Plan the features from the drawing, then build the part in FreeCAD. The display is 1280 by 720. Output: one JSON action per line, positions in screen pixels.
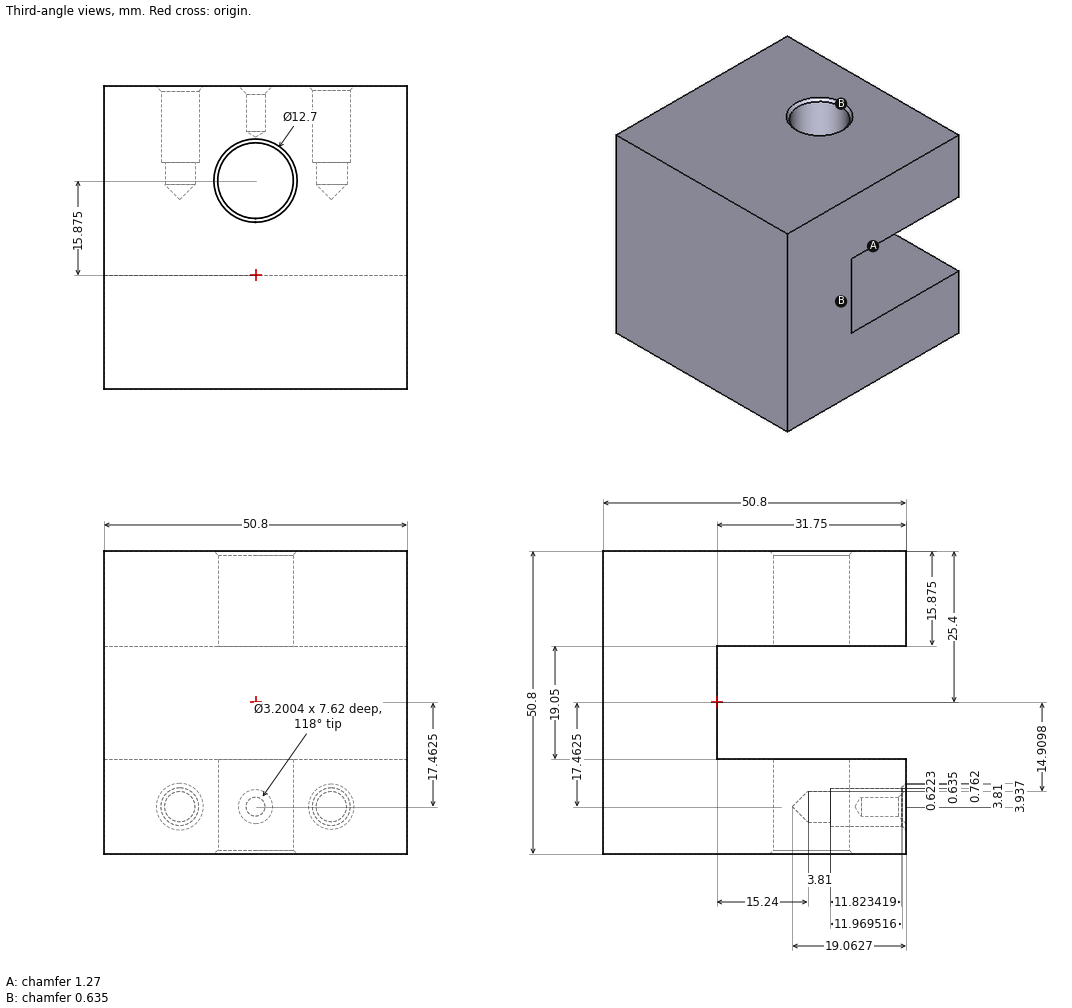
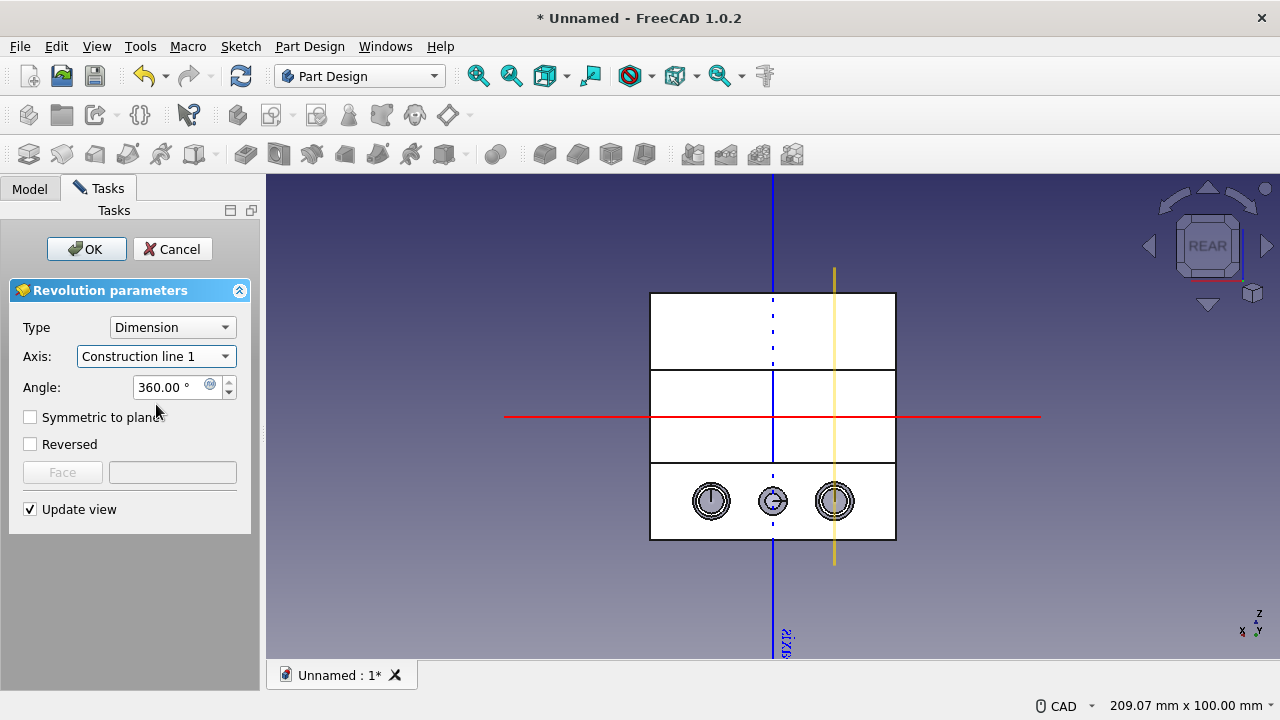
{"action": "left_click", "coordinate": [87, 249]}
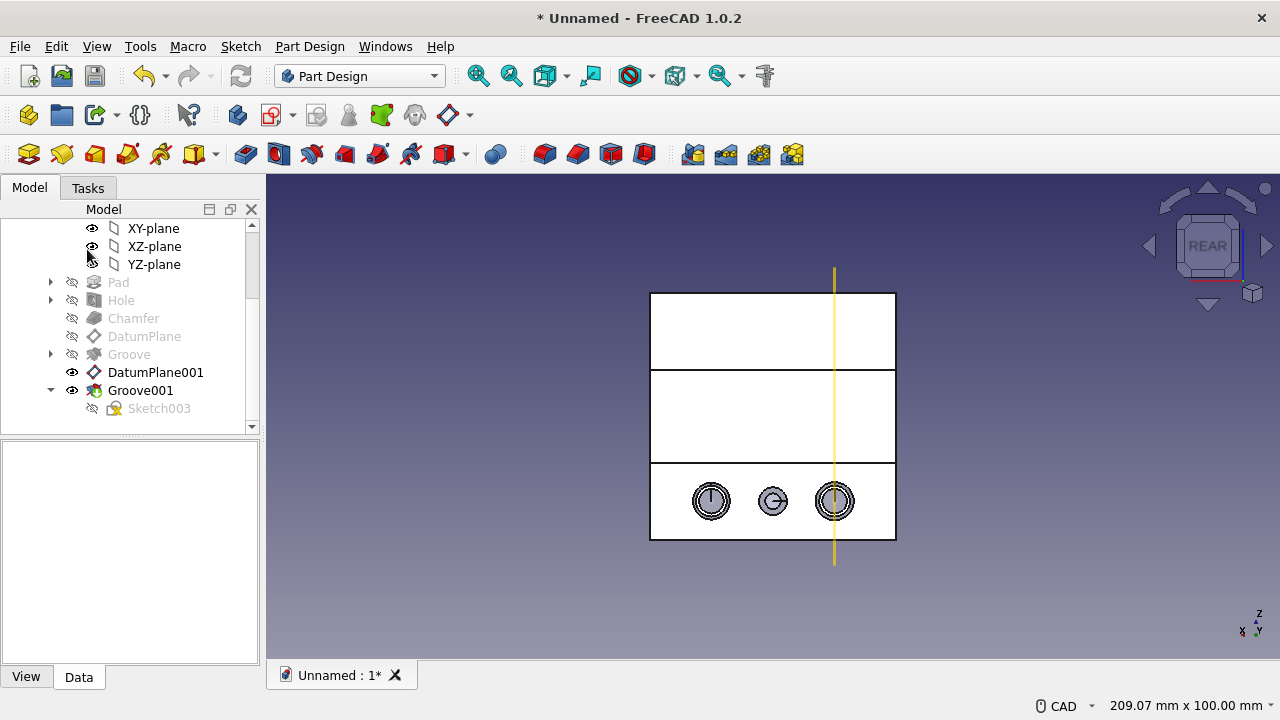
{"action": "left_click", "coordinate": [117, 372]}
{"action": "key", "text": "space"}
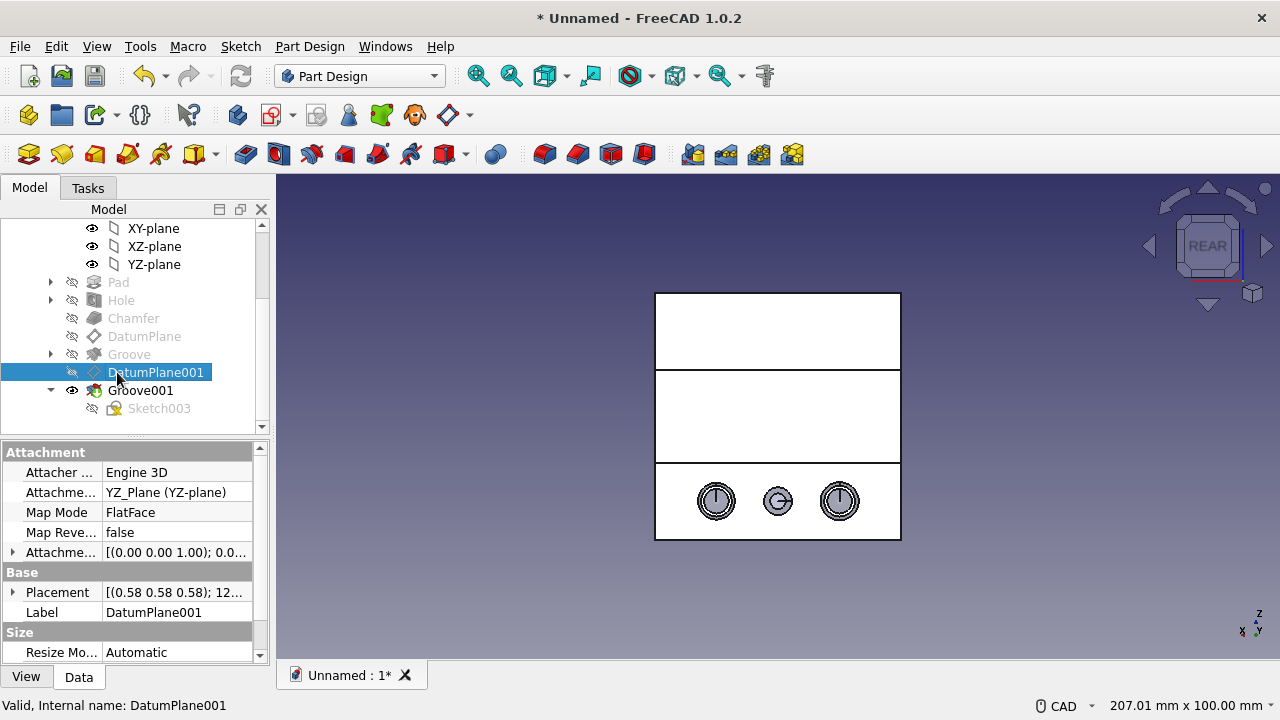
{"action": "key", "text": "0"}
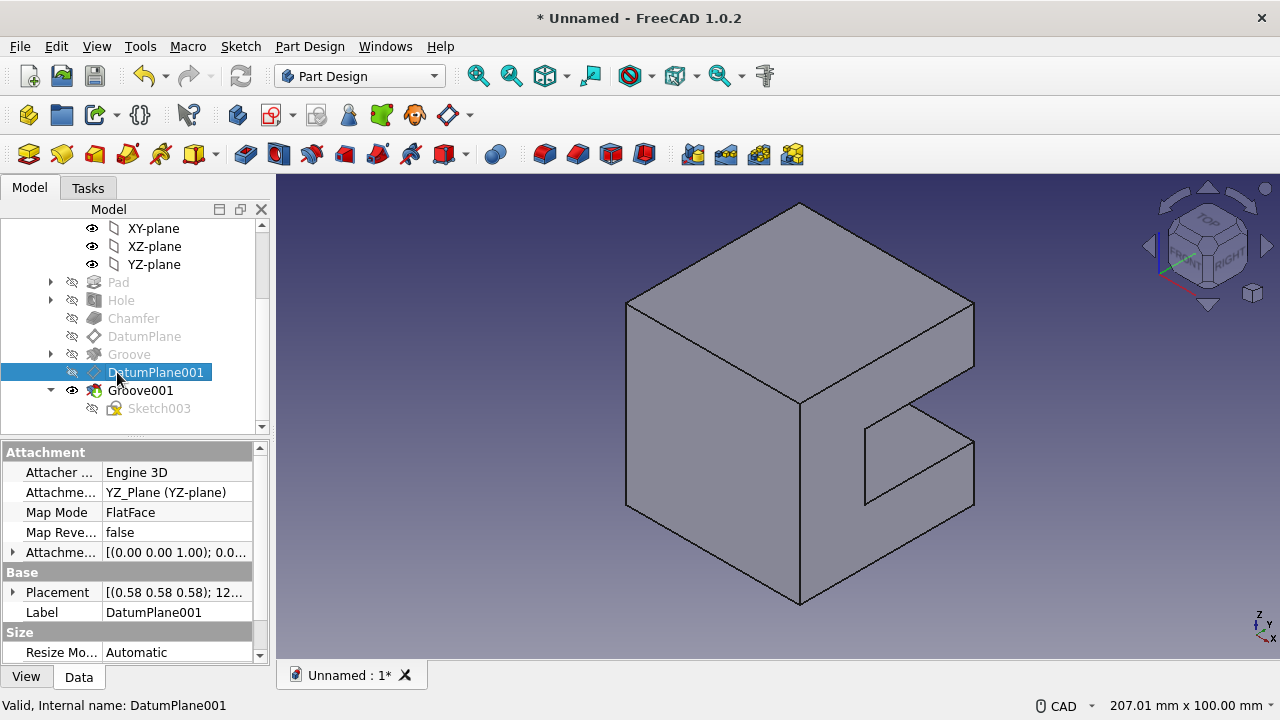
{"action": "left_click", "coordinate": [800, 302]}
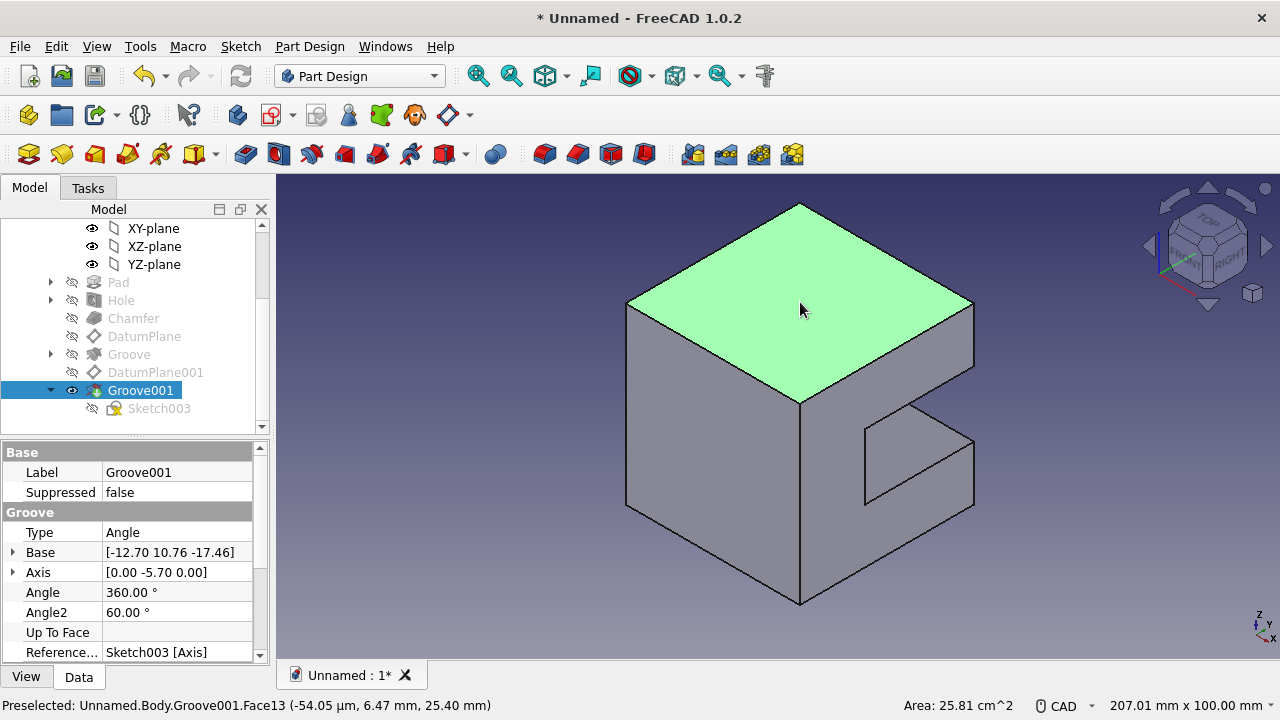
{"action": "left_click", "coordinate": [270, 116]}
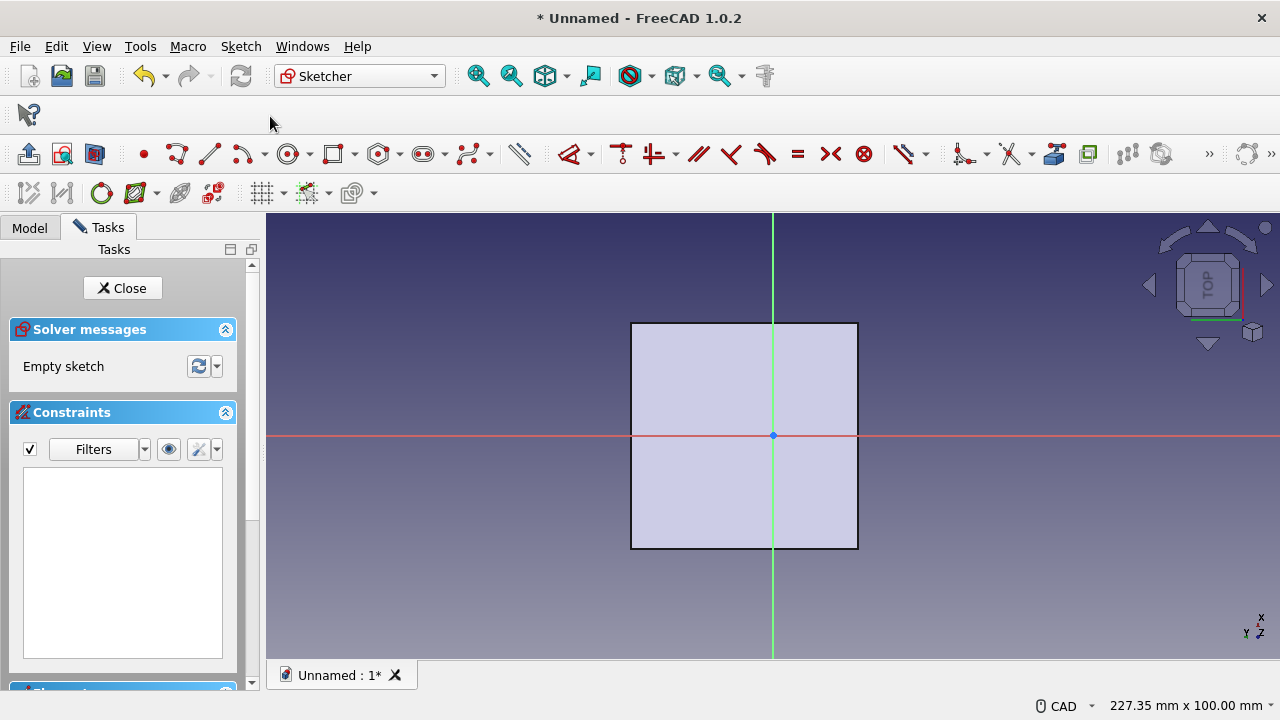
{"action": "scroll", "coordinate": [728, 436], "scroll_direction": "up", "scroll_amount": 8}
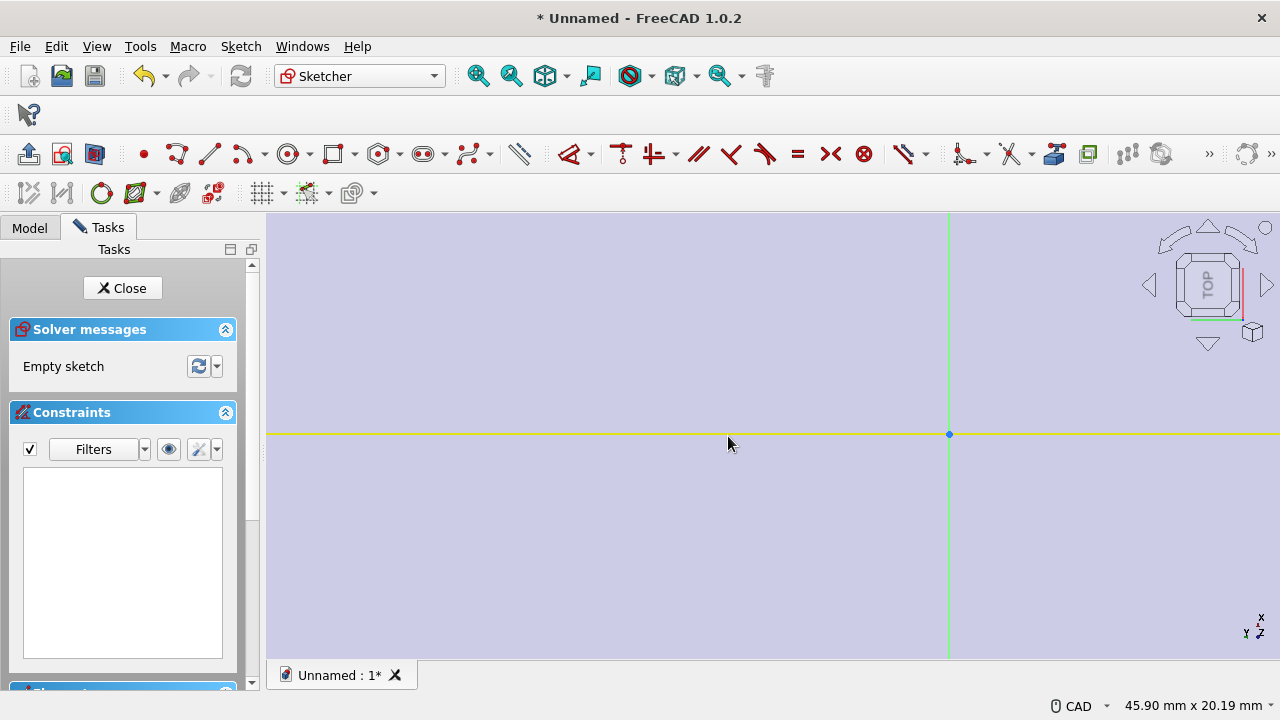
{"action": "left_click", "coordinate": [288, 154]}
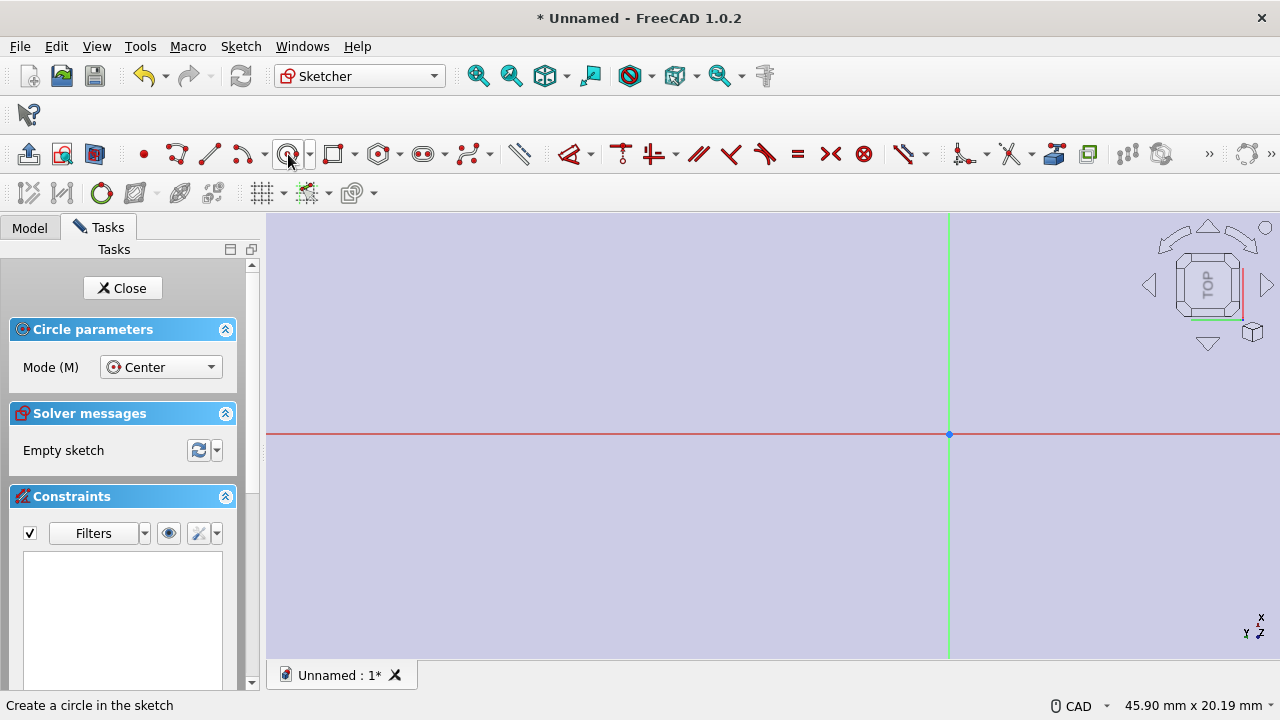
{"action": "left_click", "coordinate": [598, 434]}
{"action": "left_click", "coordinate": [698, 335]}
{"action": "key", "text": "Escape"}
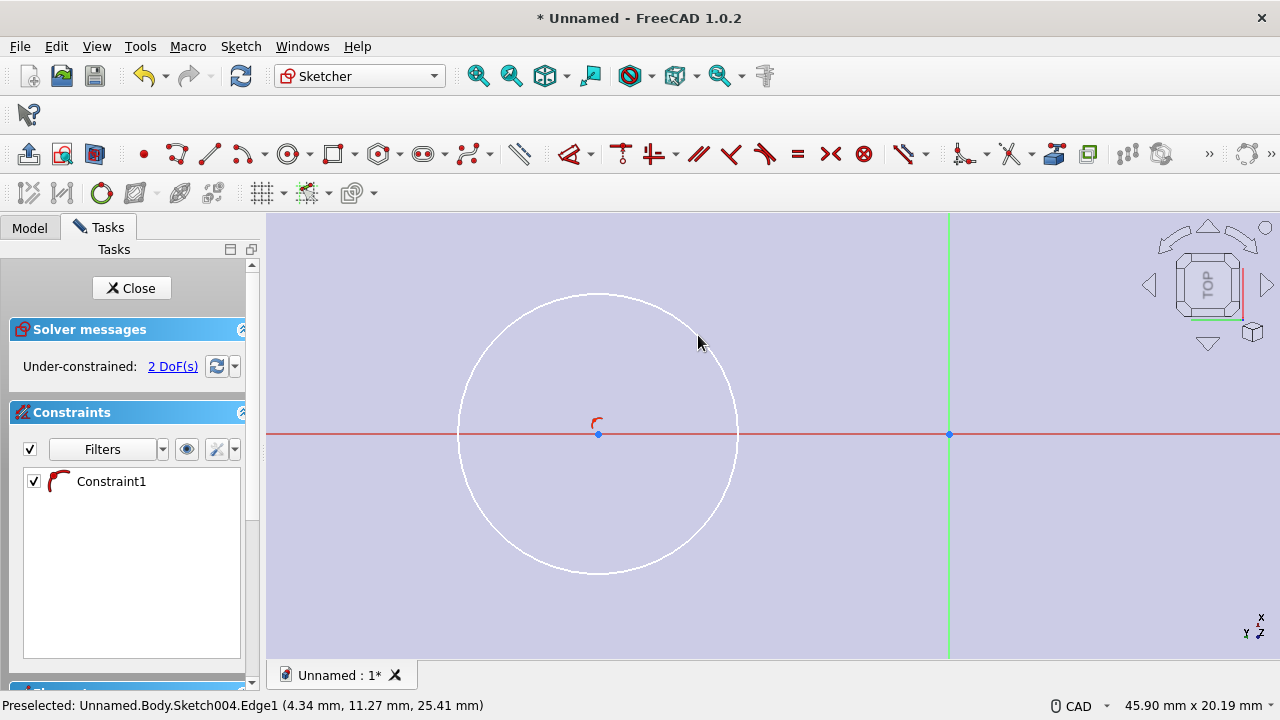
{"action": "left_click", "coordinate": [568, 154]}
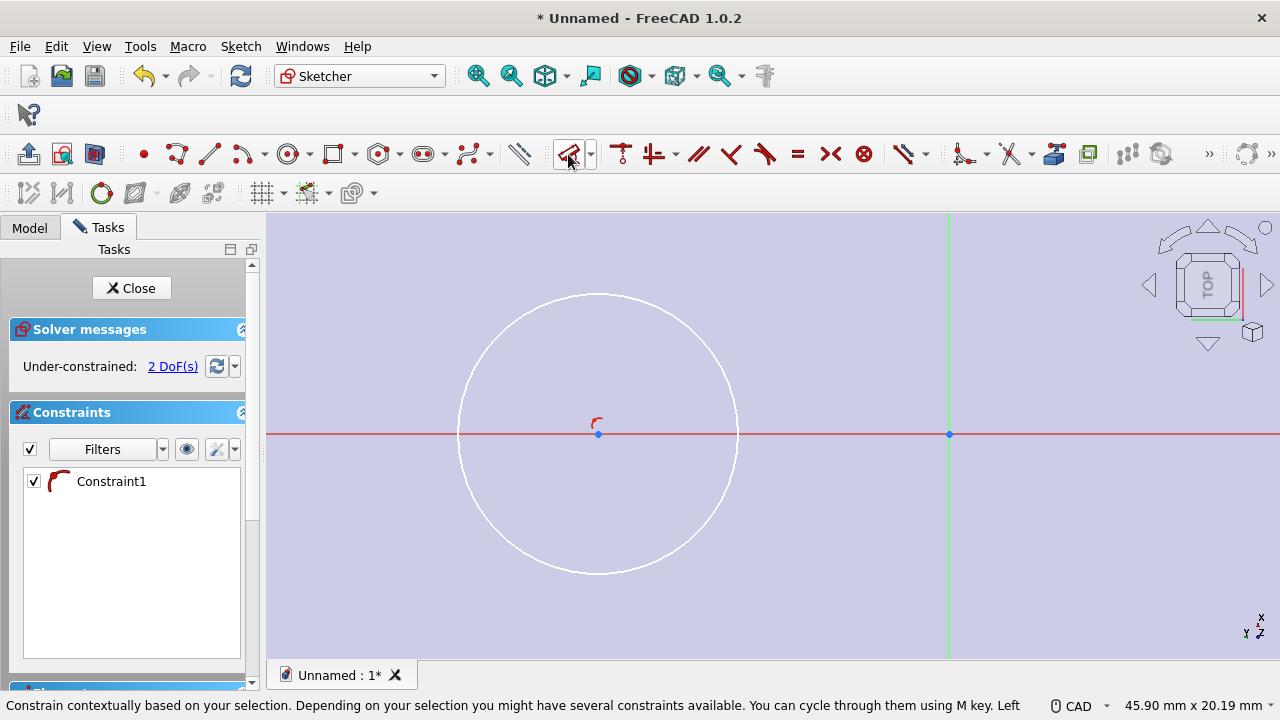
{"action": "left_click", "coordinate": [697, 335]}
{"action": "left_click", "coordinate": [720, 312]}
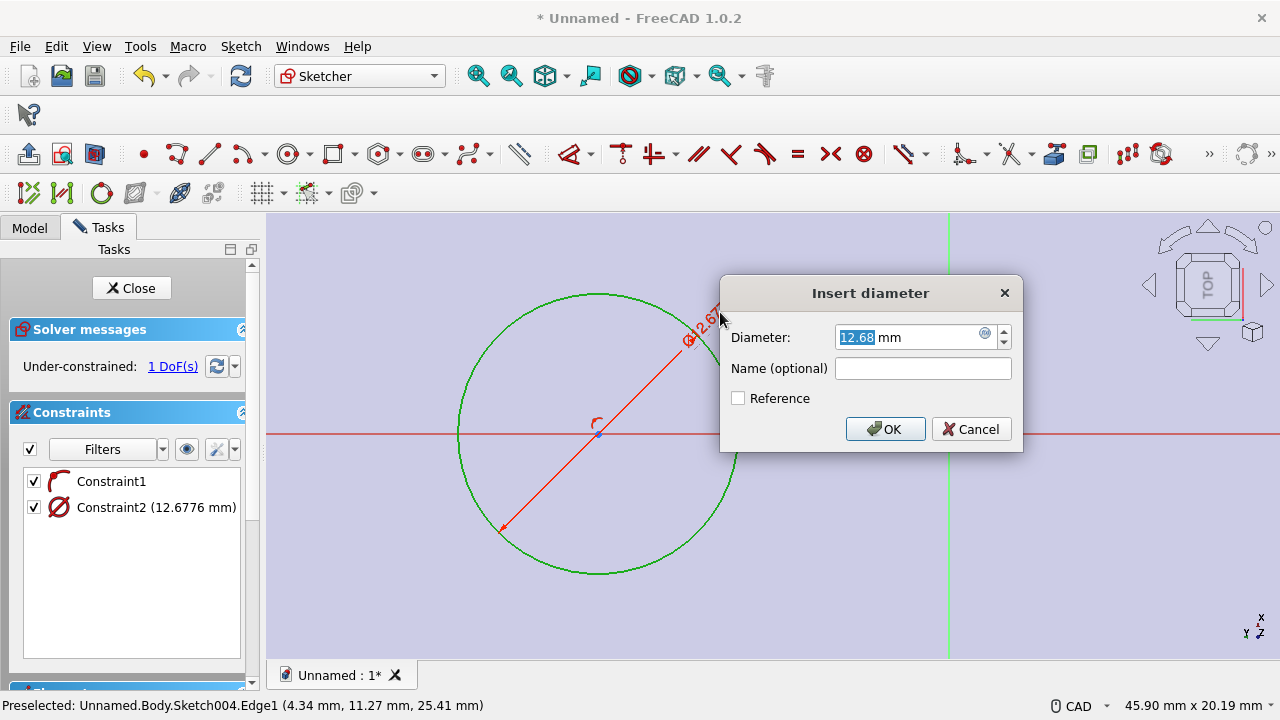
{"action": "type", "text": "12.7"}
{"action": "key", "text": "Return"}